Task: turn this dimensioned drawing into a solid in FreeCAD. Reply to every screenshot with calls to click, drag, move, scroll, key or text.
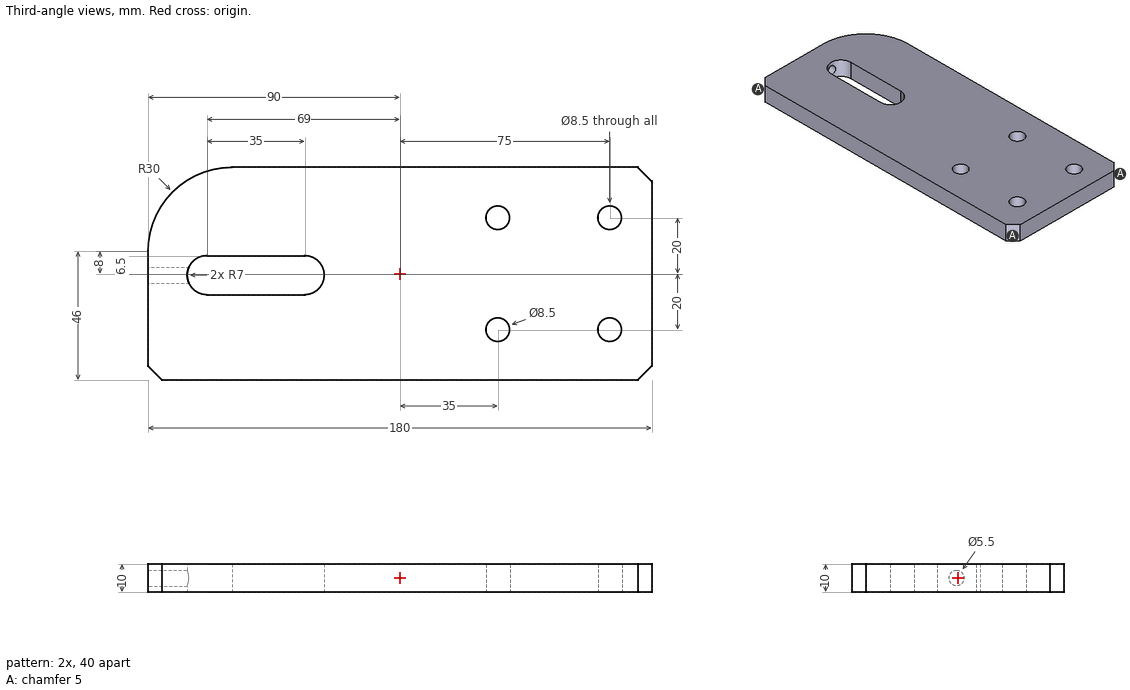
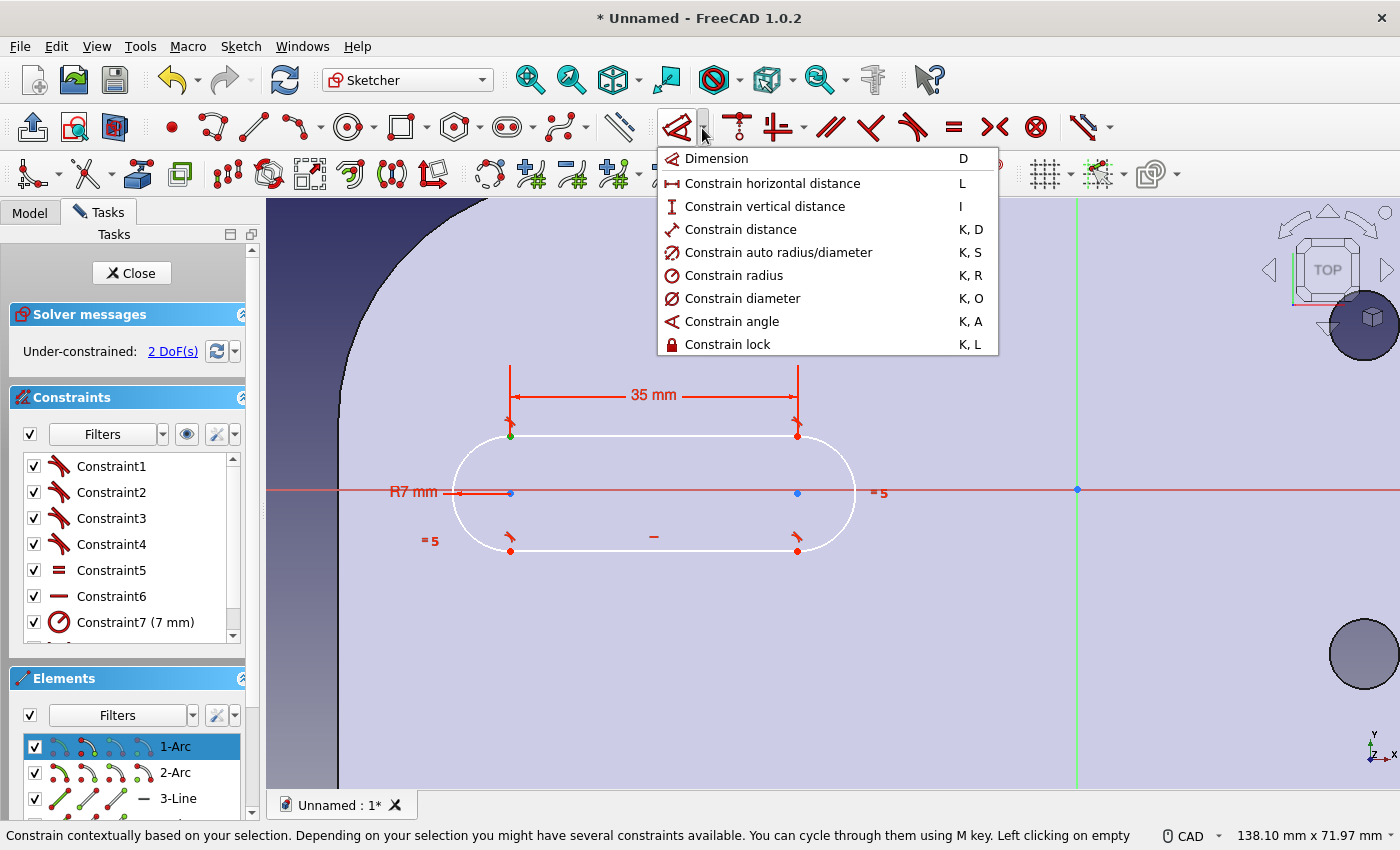
click(828, 184)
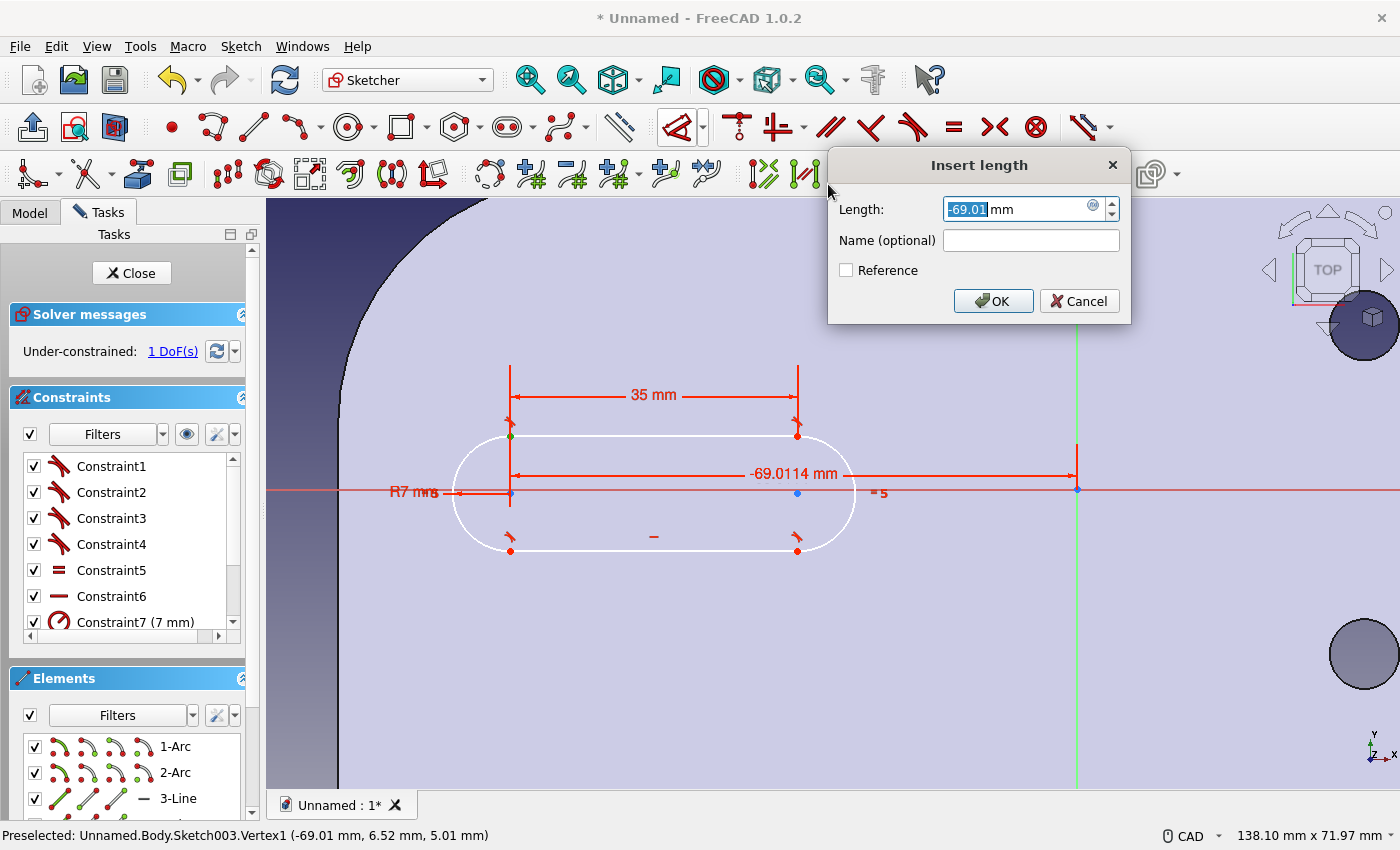
text(-69)
key(Return)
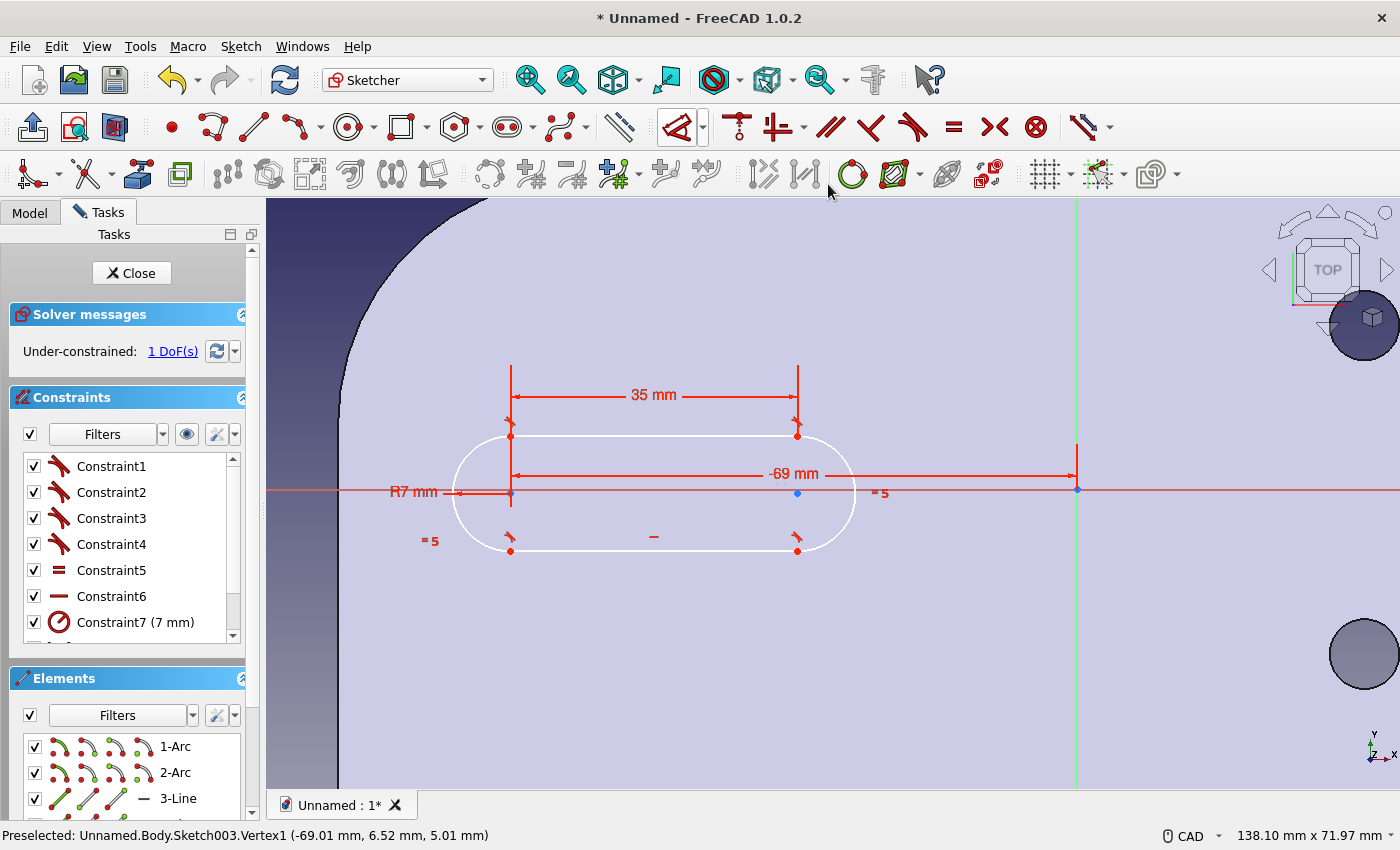
click(511, 436)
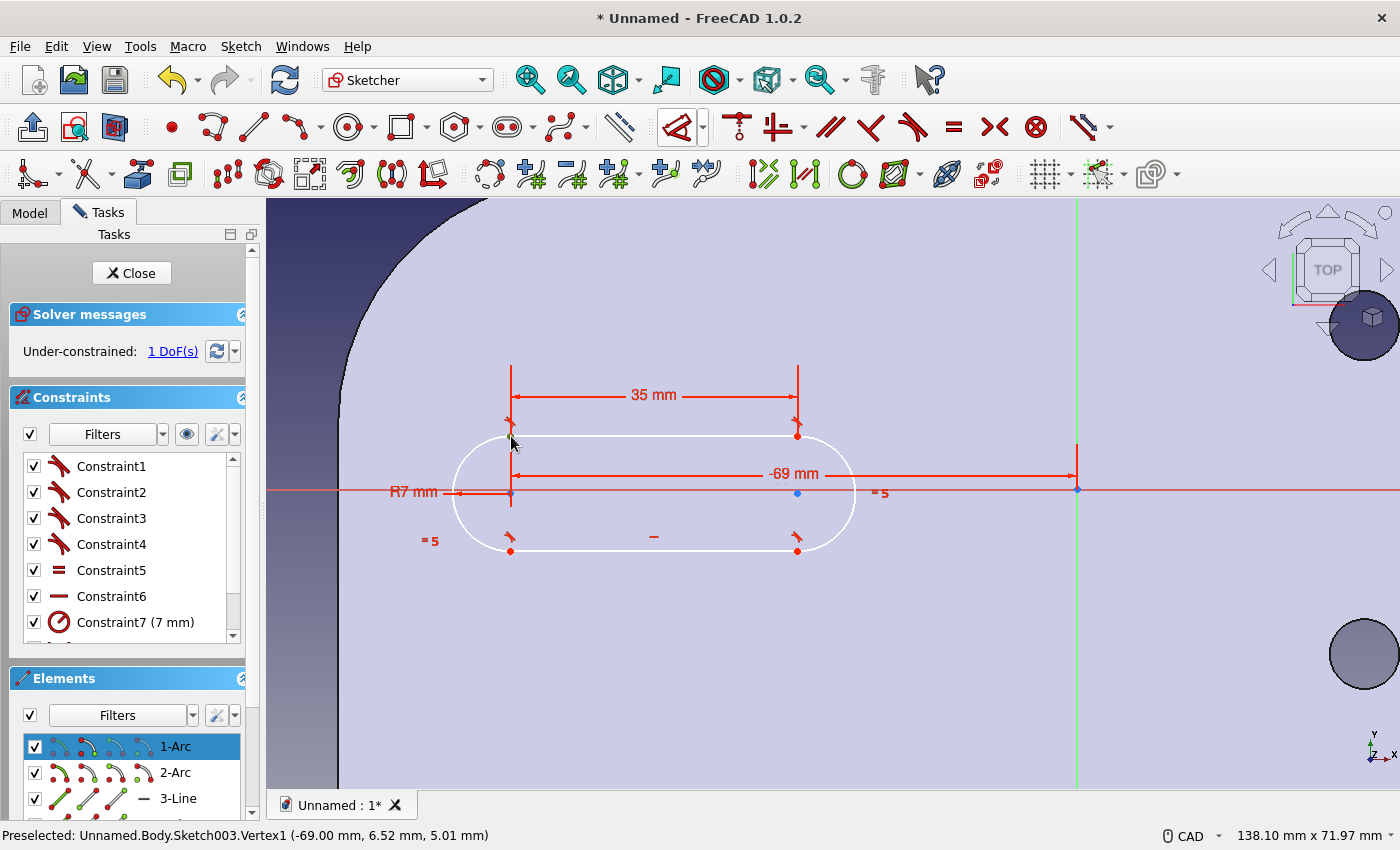
key(i)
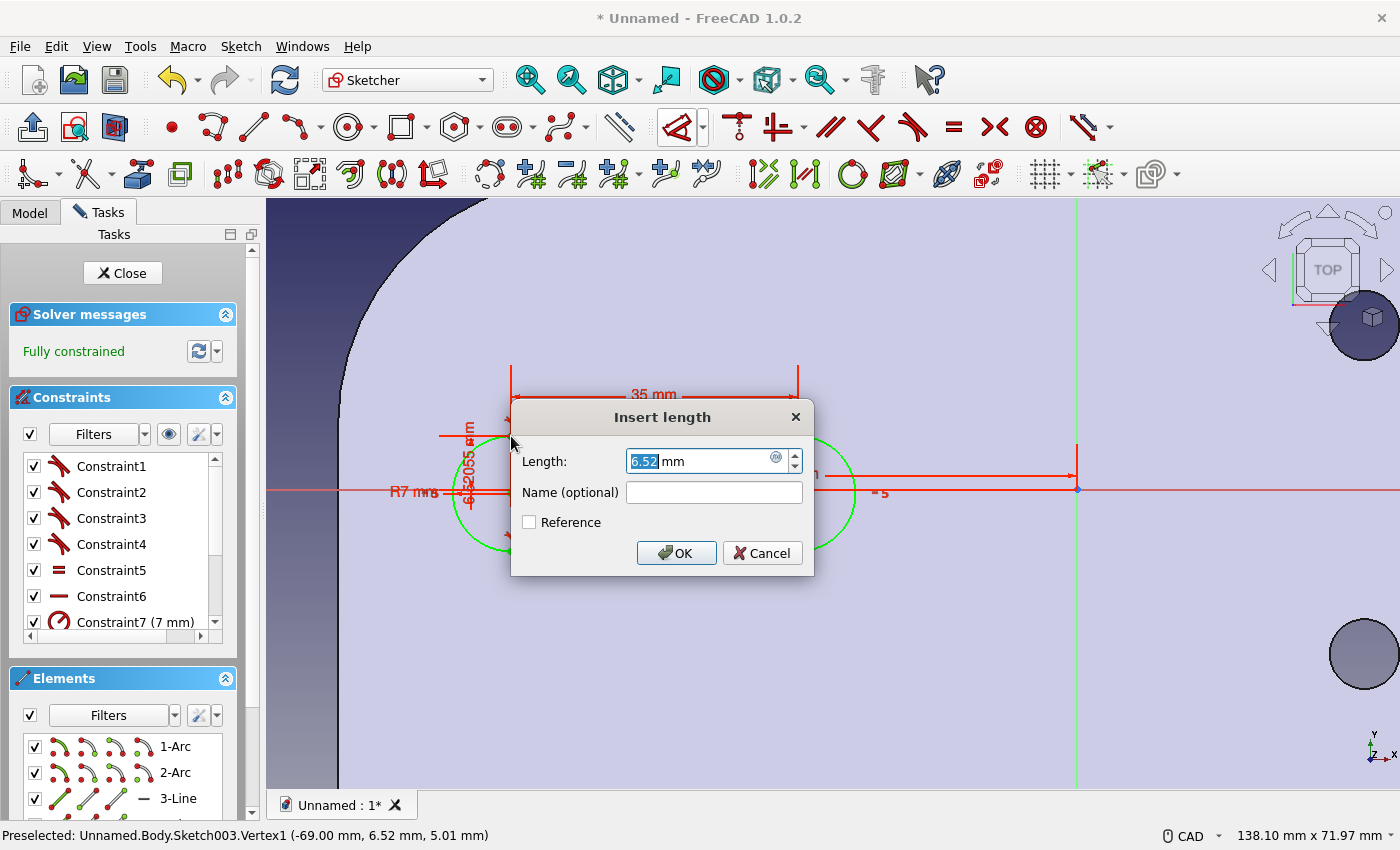
text(6.5)
key(Return)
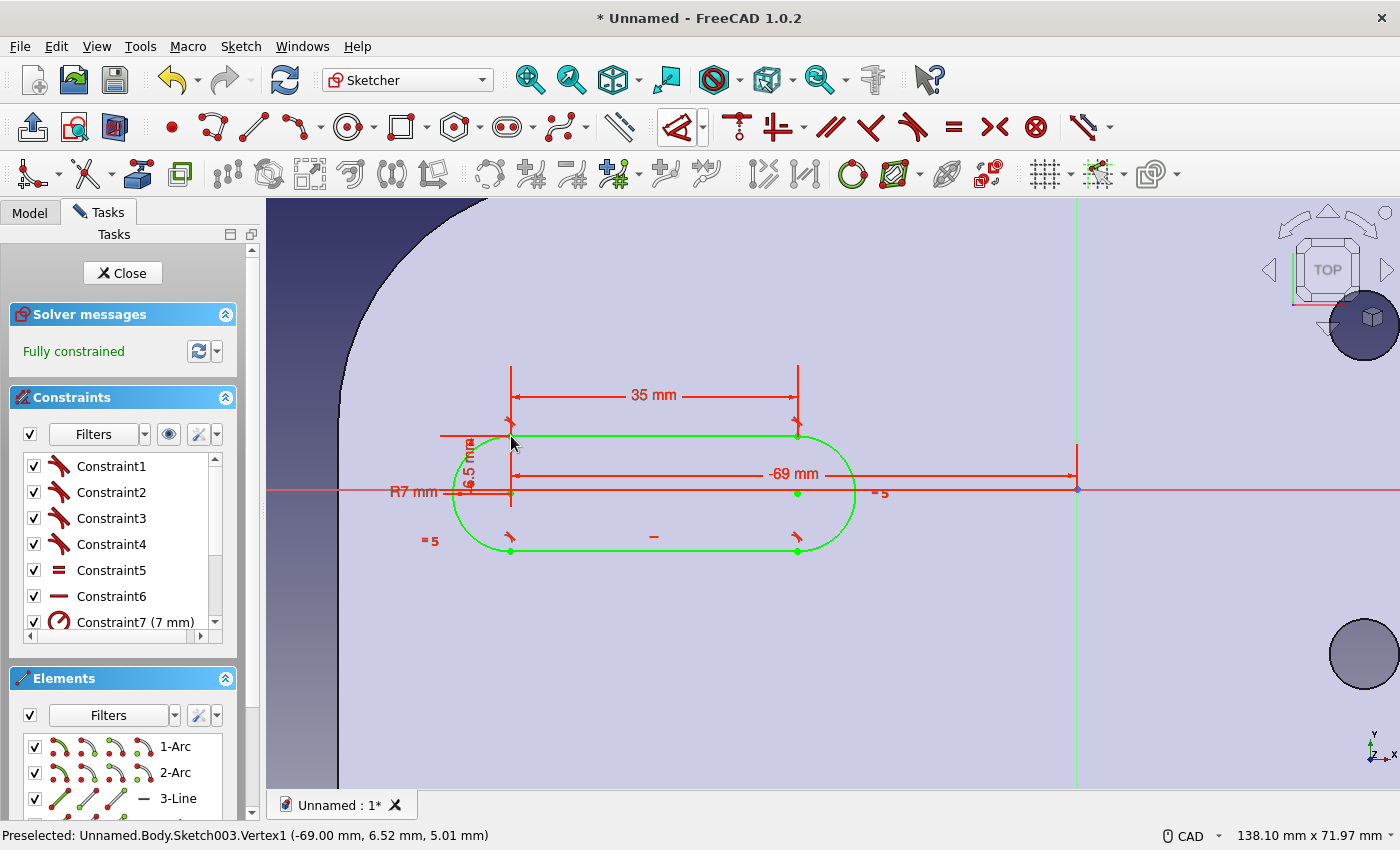
click(123, 273)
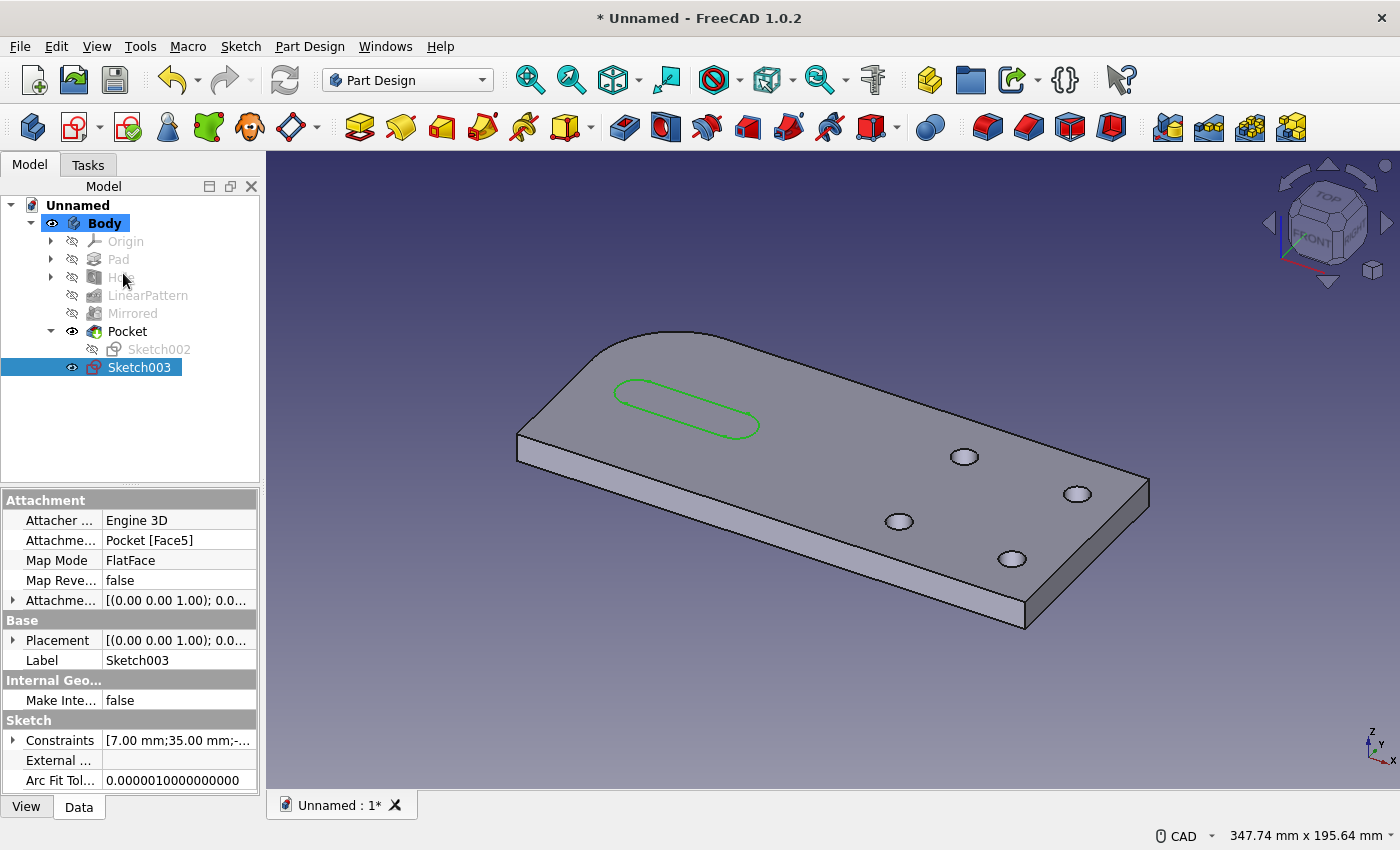
click(625, 128)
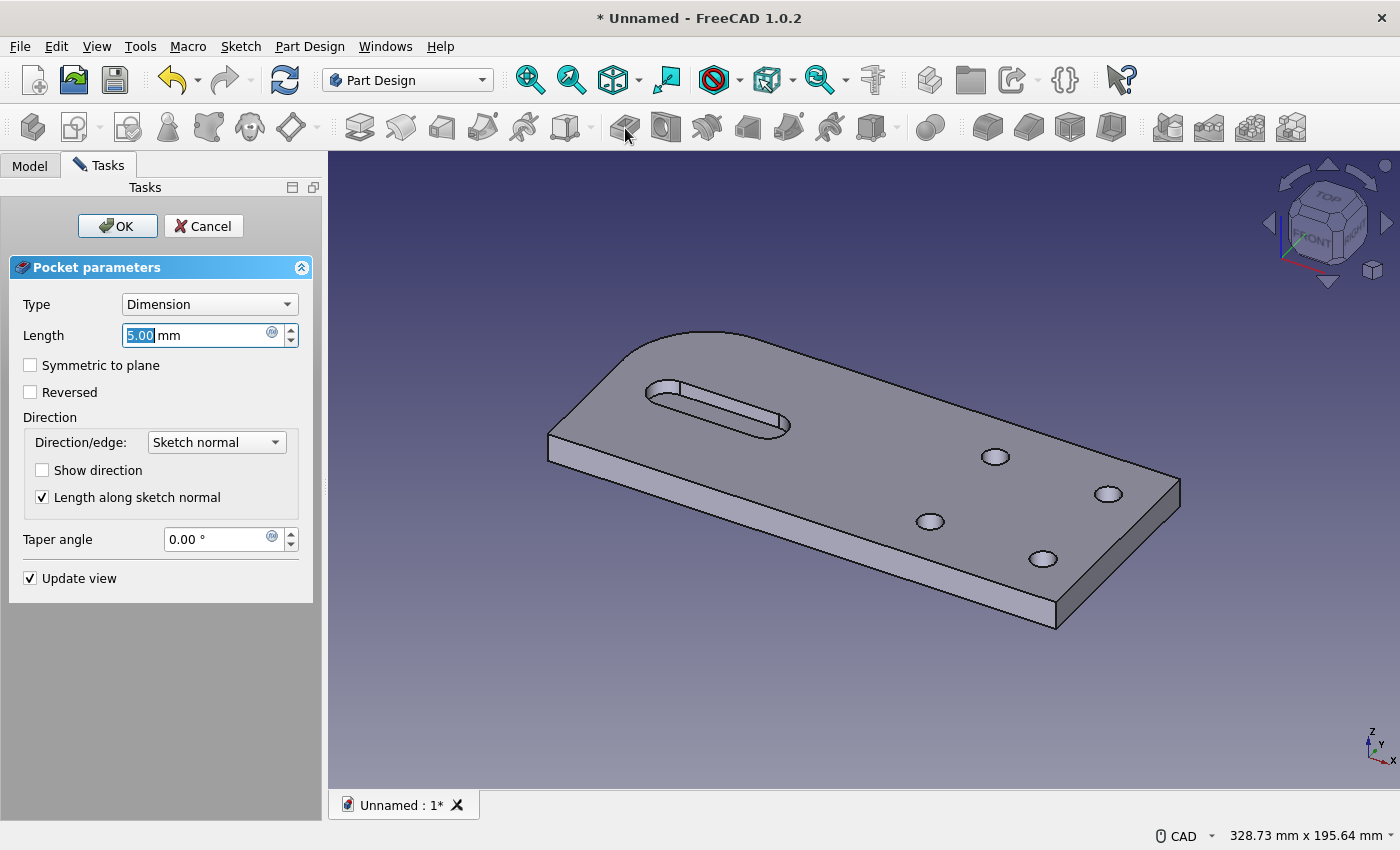
text(10)
key(Tab)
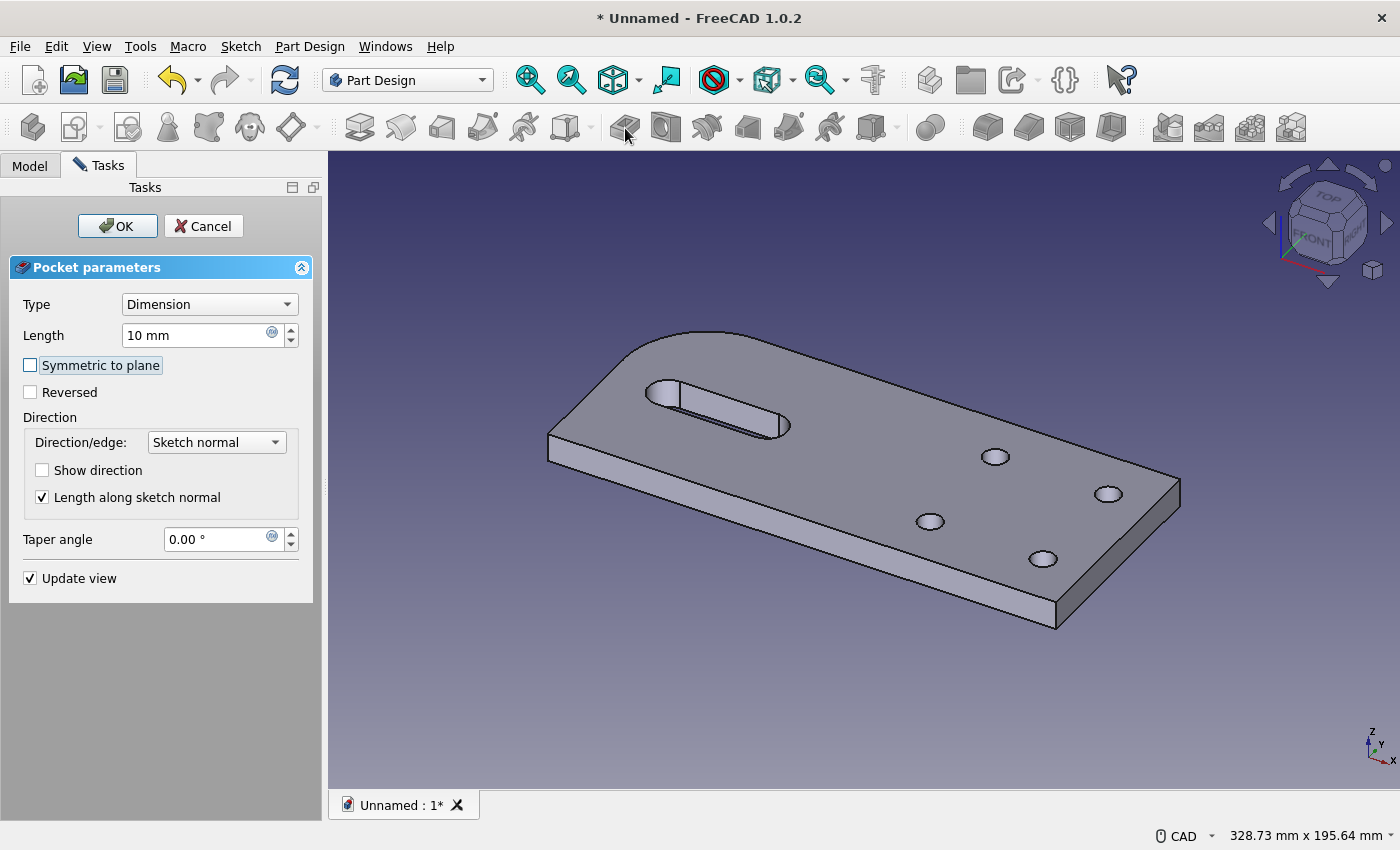
click(118, 226)